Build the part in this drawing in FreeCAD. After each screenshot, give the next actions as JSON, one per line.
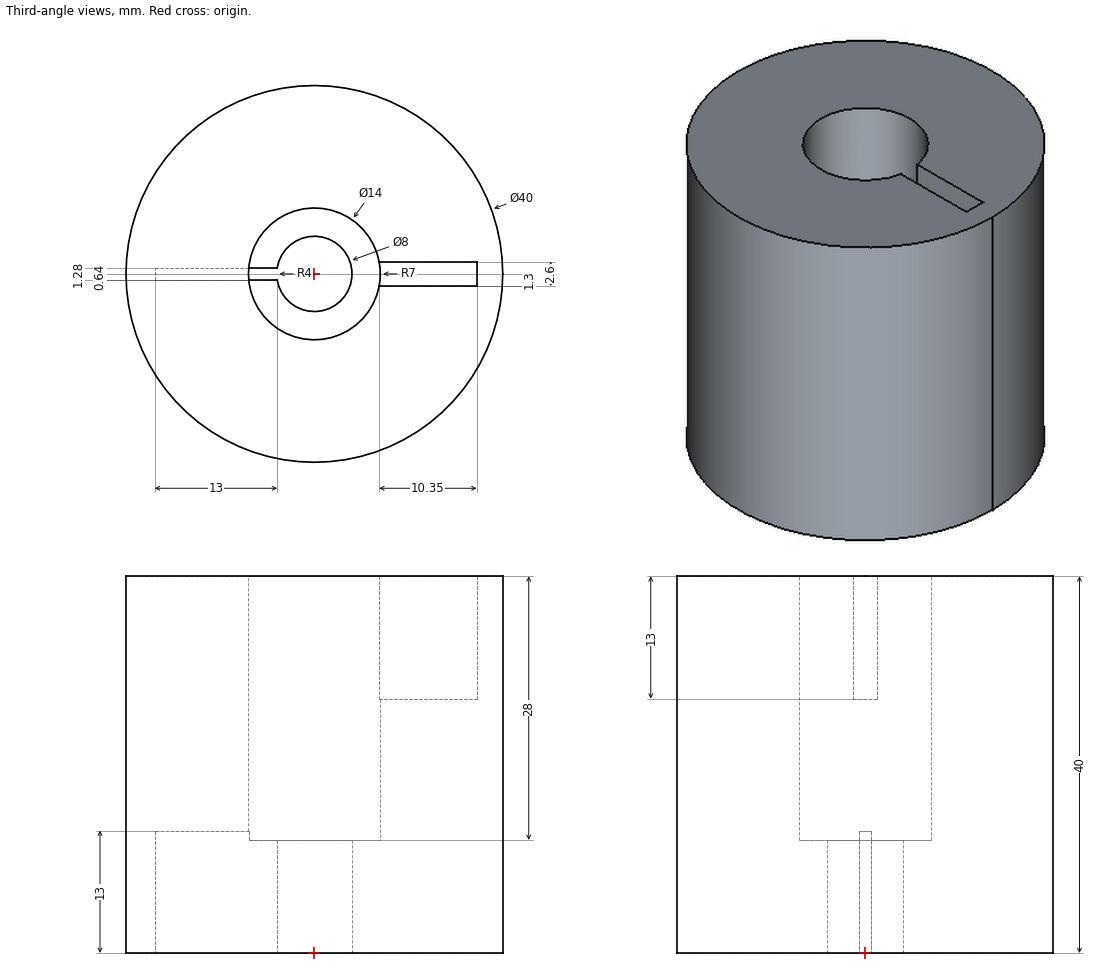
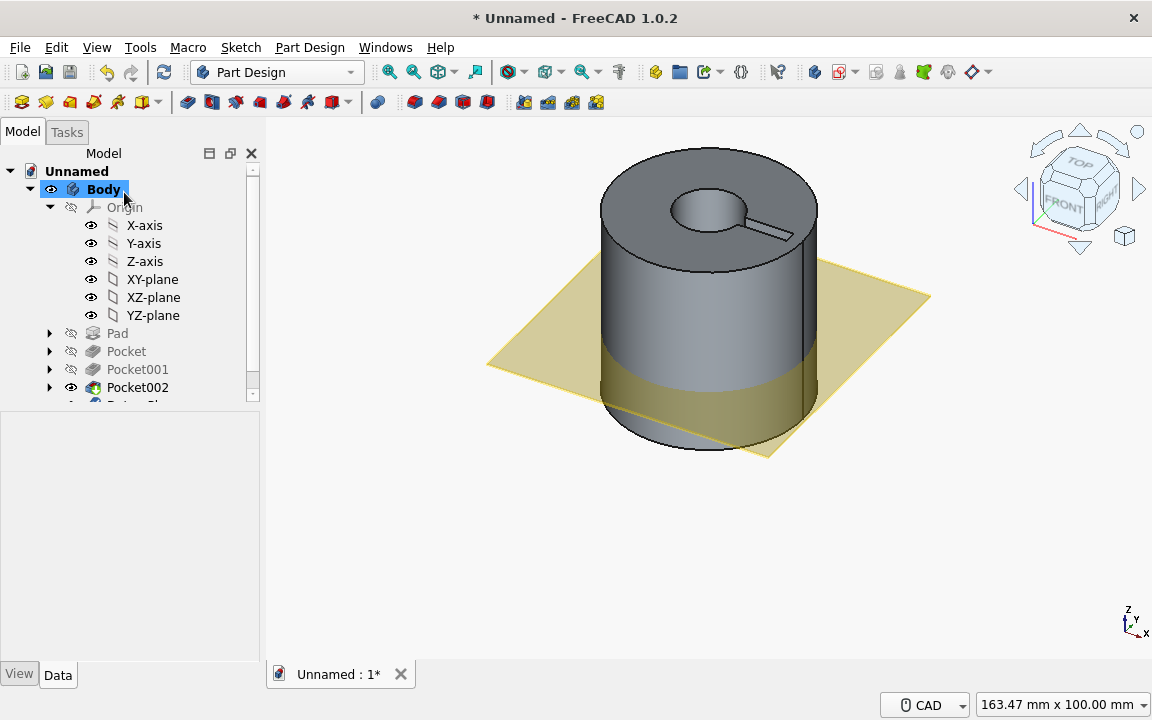
{"action": "scroll", "coordinate": [100, 275], "scroll_direction": "down", "scroll_amount": 3}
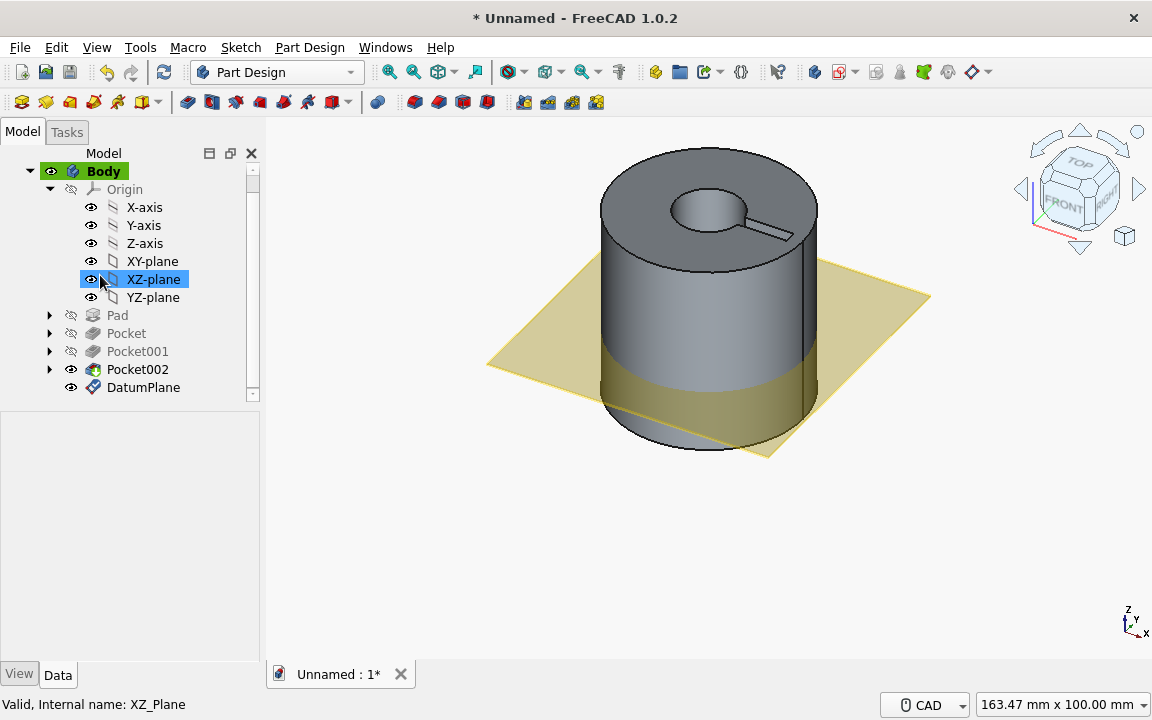
{"action": "left_click", "coordinate": [116, 387]}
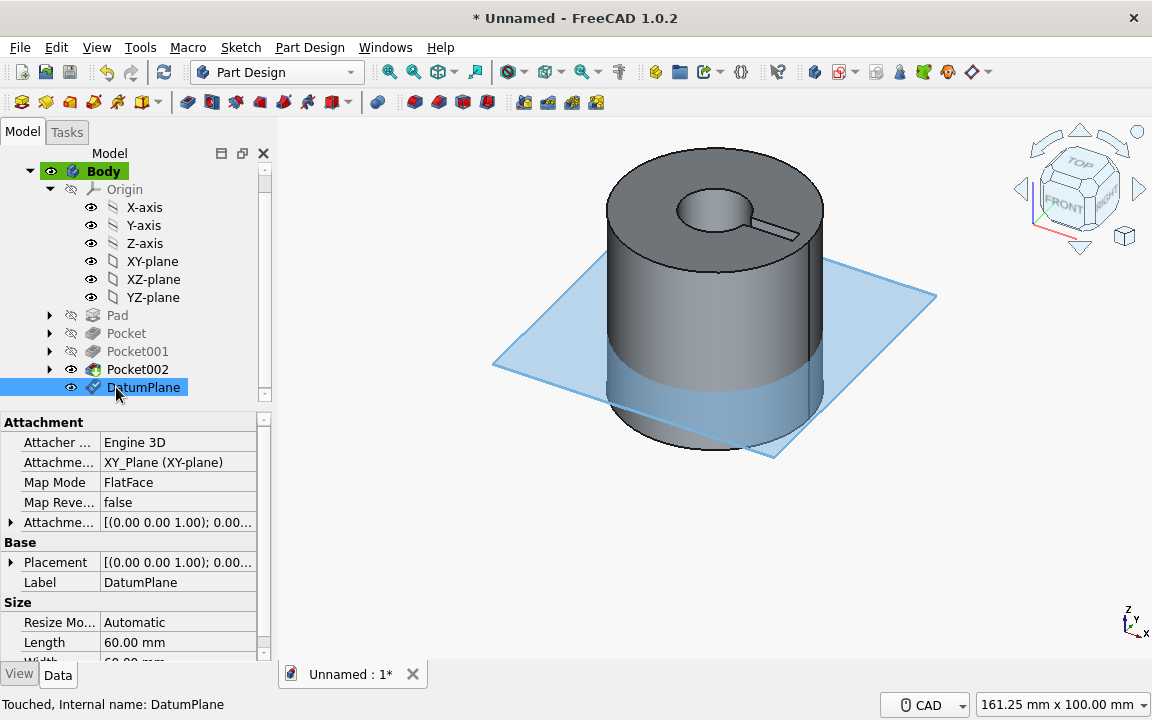
{"action": "left_click", "coordinate": [840, 72]}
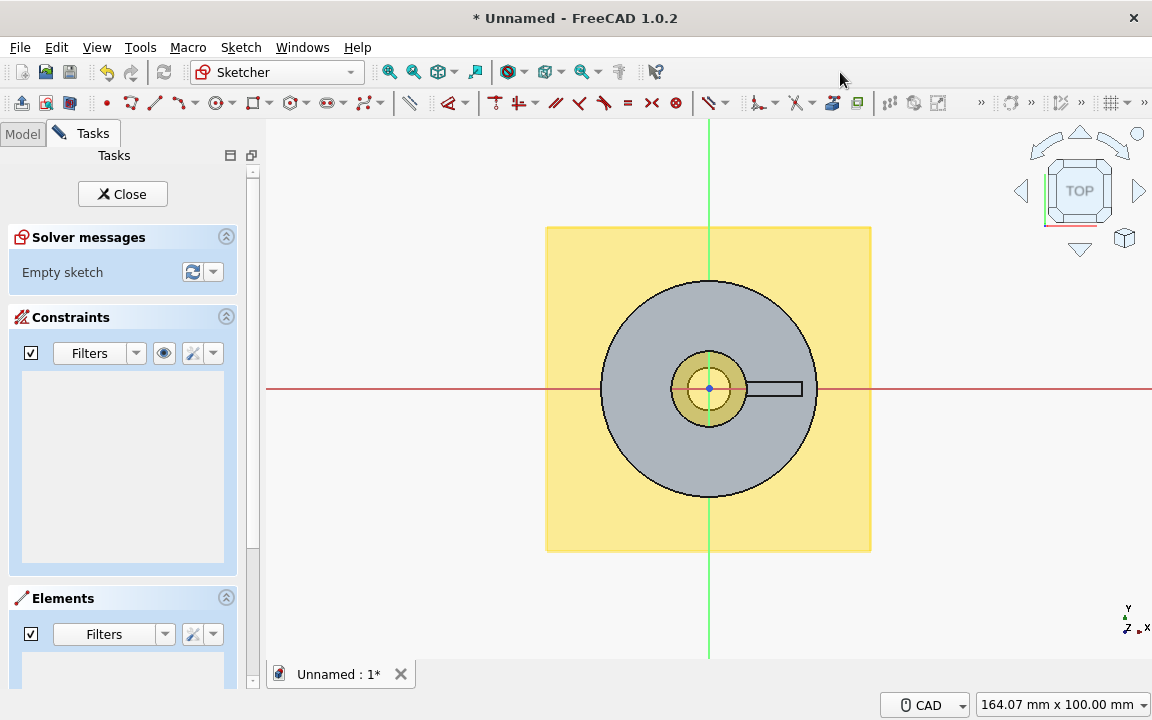
{"action": "key", "text": "q s"}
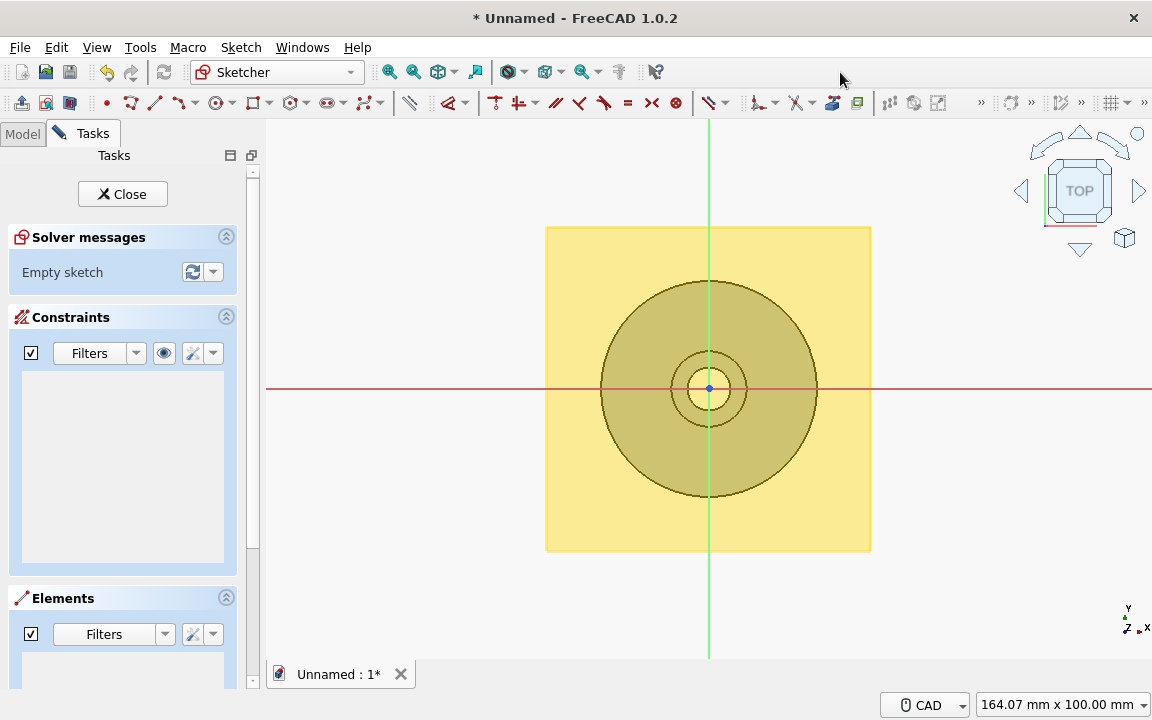
{"action": "scroll", "coordinate": [669, 389], "scroll_direction": "up", "scroll_amount": 8}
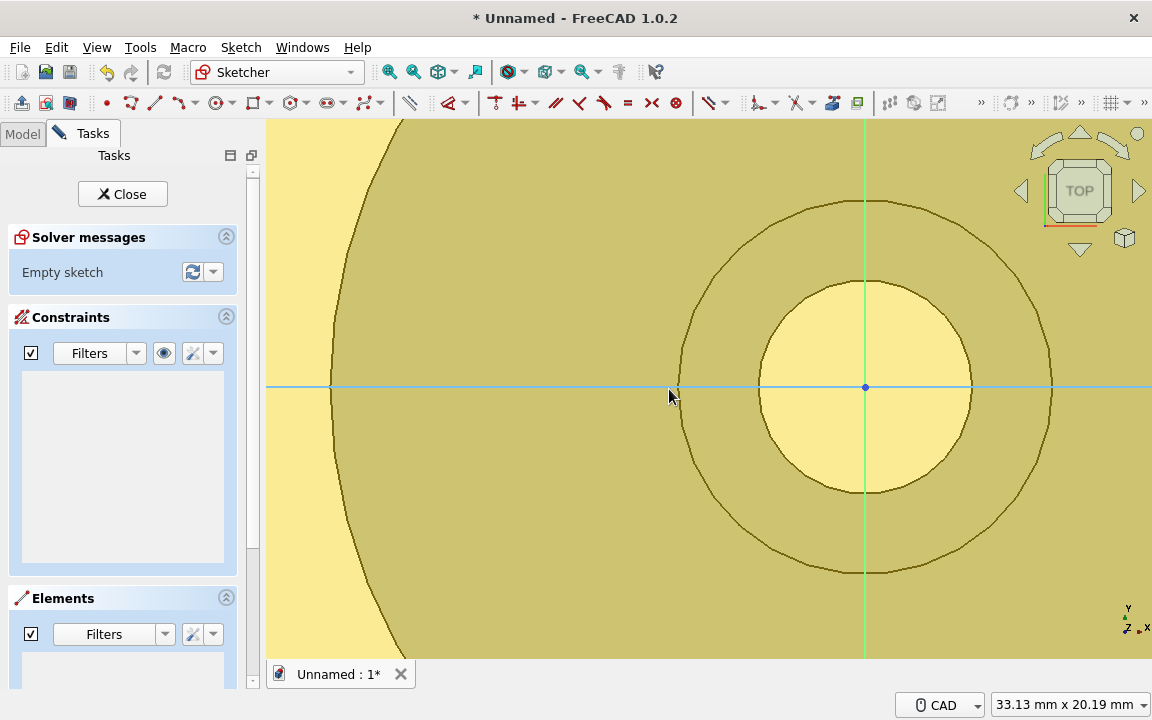
{"action": "key", "text": "g m"}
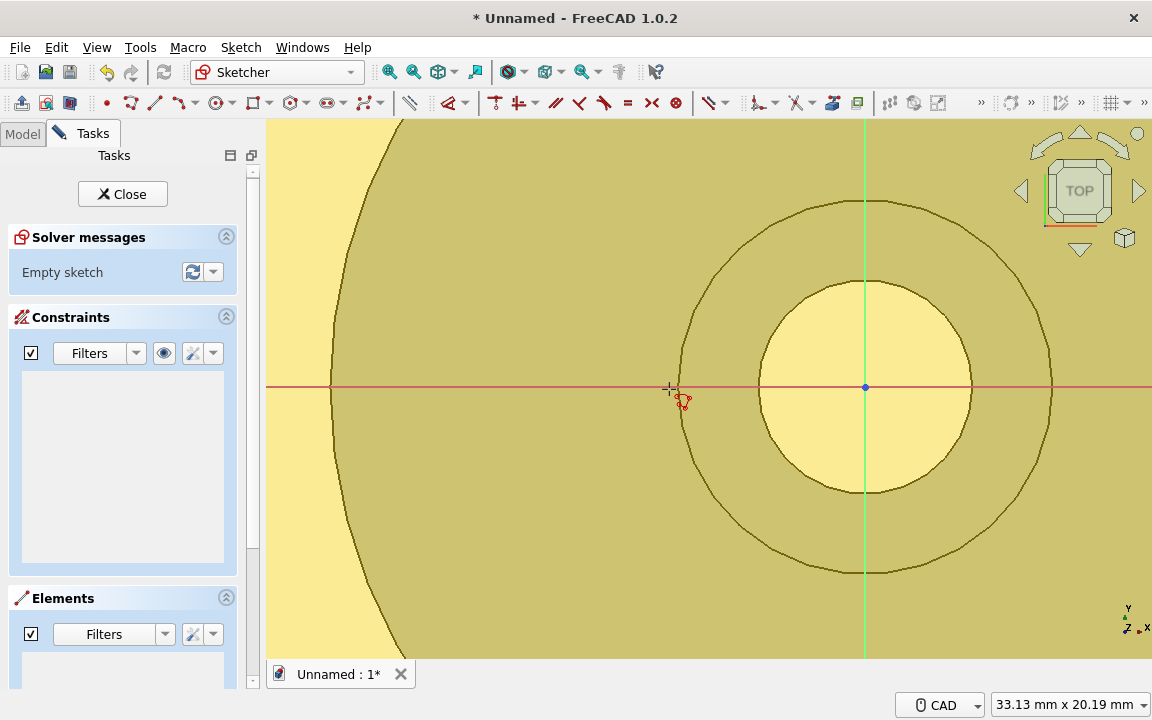
{"action": "left_click", "coordinate": [760, 404]}
{"action": "left_click", "coordinate": [412, 404]}
{"action": "left_click", "coordinate": [412, 370]}
{"action": "left_click", "coordinate": [760, 370]}
{"action": "right_click", "coordinate": [760, 370]}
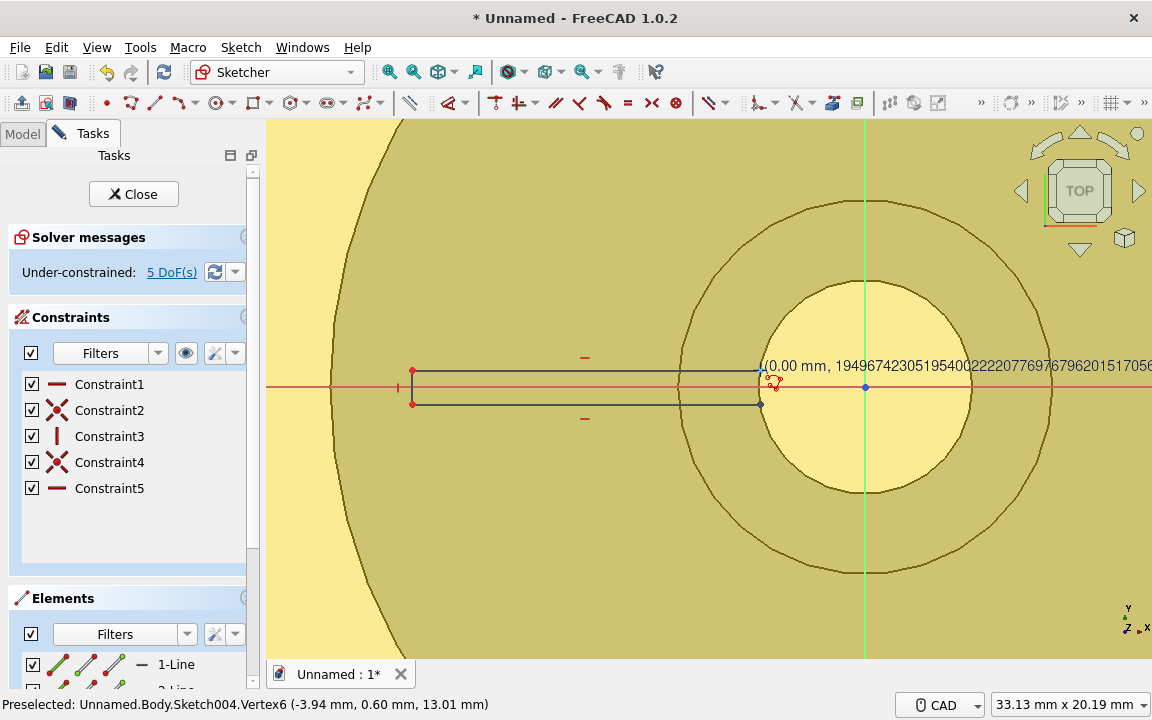
{"action": "key", "text": "g 3 a"}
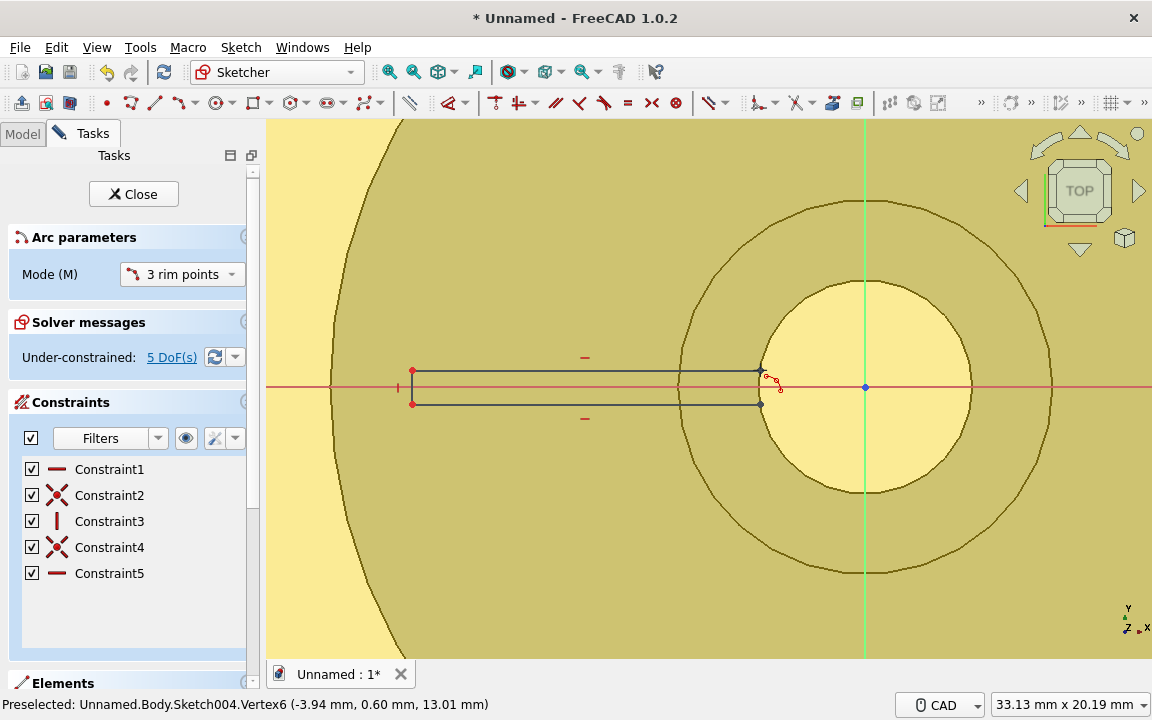
{"action": "left_click", "coordinate": [760, 371]}
{"action": "left_click", "coordinate": [760, 405]}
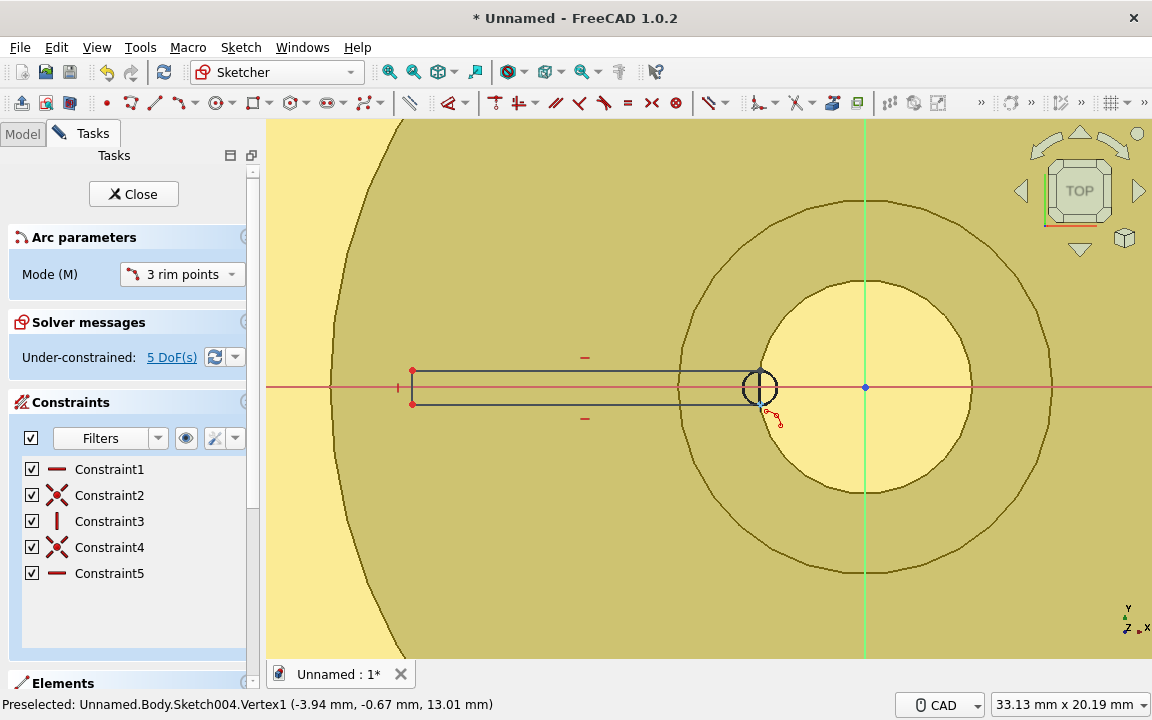
{"action": "scroll", "coordinate": [758, 384], "scroll_direction": "up", "scroll_amount": 13}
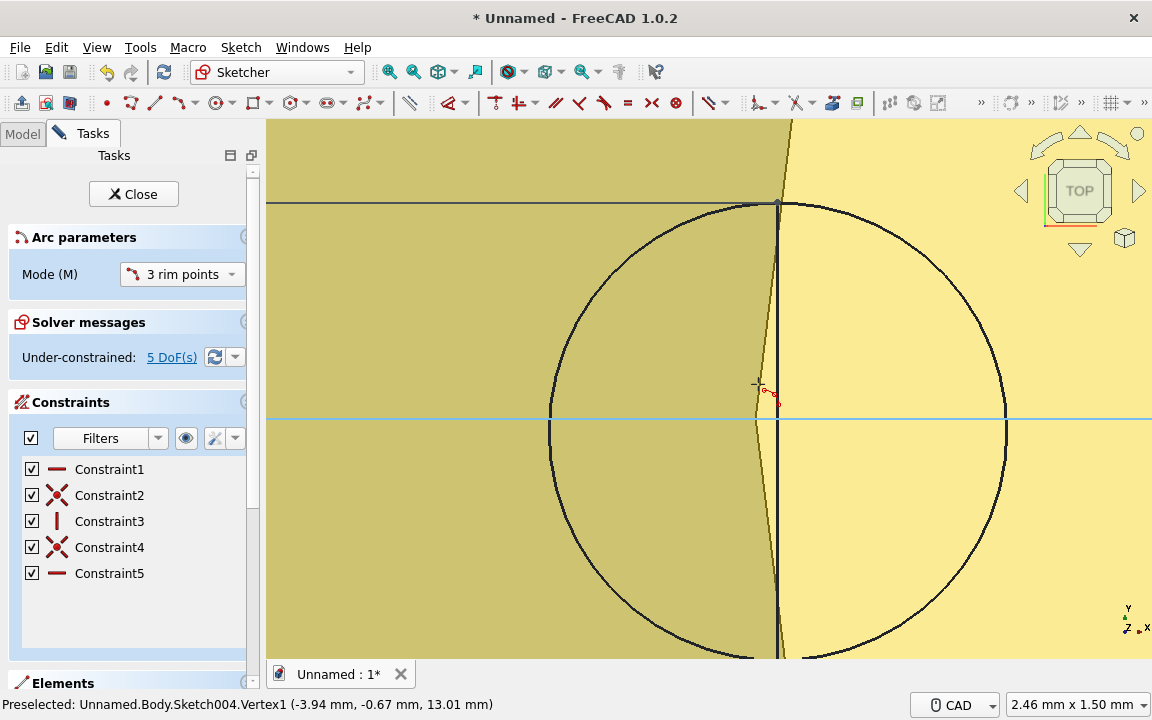
{"action": "left_click", "coordinate": [756, 372]}
{"action": "key", "text": "Escape"}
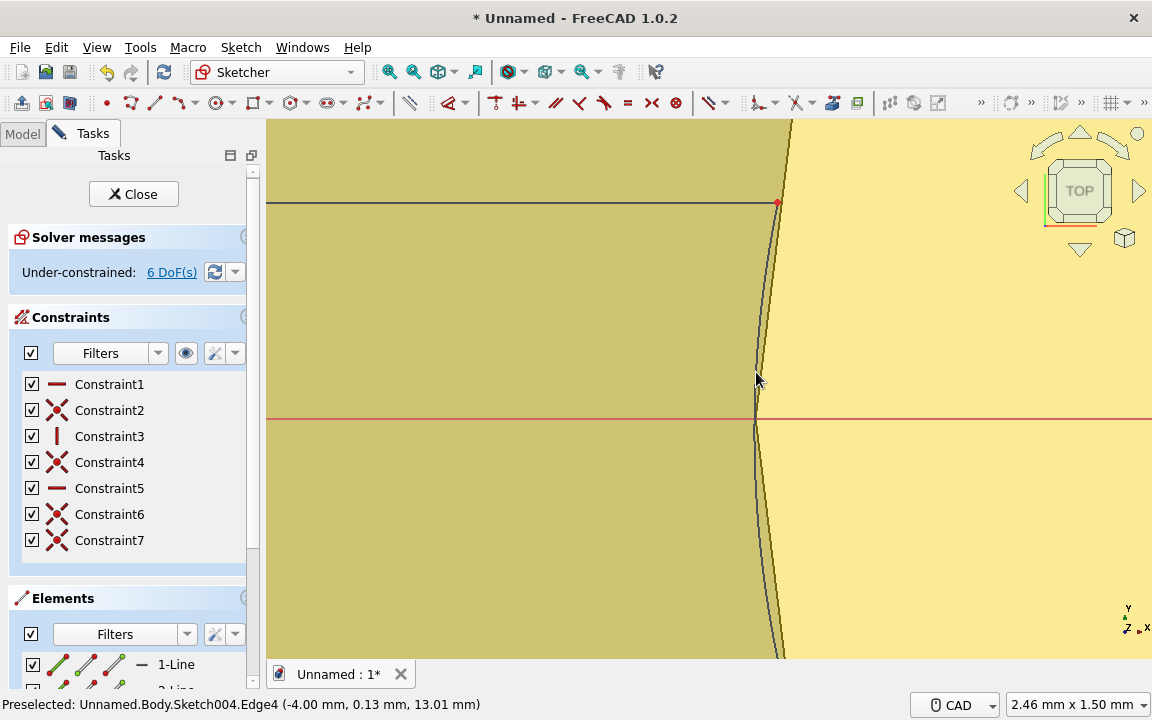
{"action": "scroll", "coordinate": [761, 387], "scroll_direction": "down", "scroll_amount": 13}